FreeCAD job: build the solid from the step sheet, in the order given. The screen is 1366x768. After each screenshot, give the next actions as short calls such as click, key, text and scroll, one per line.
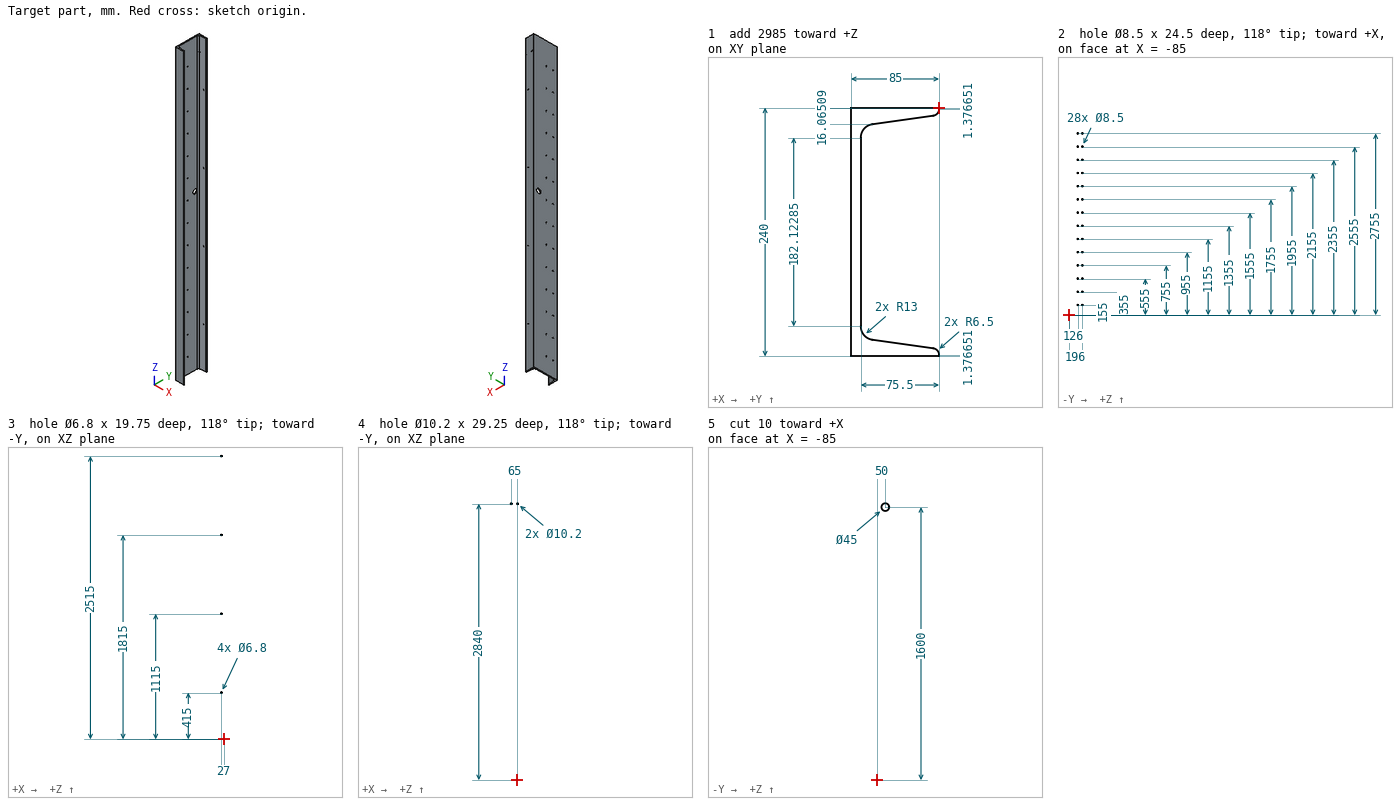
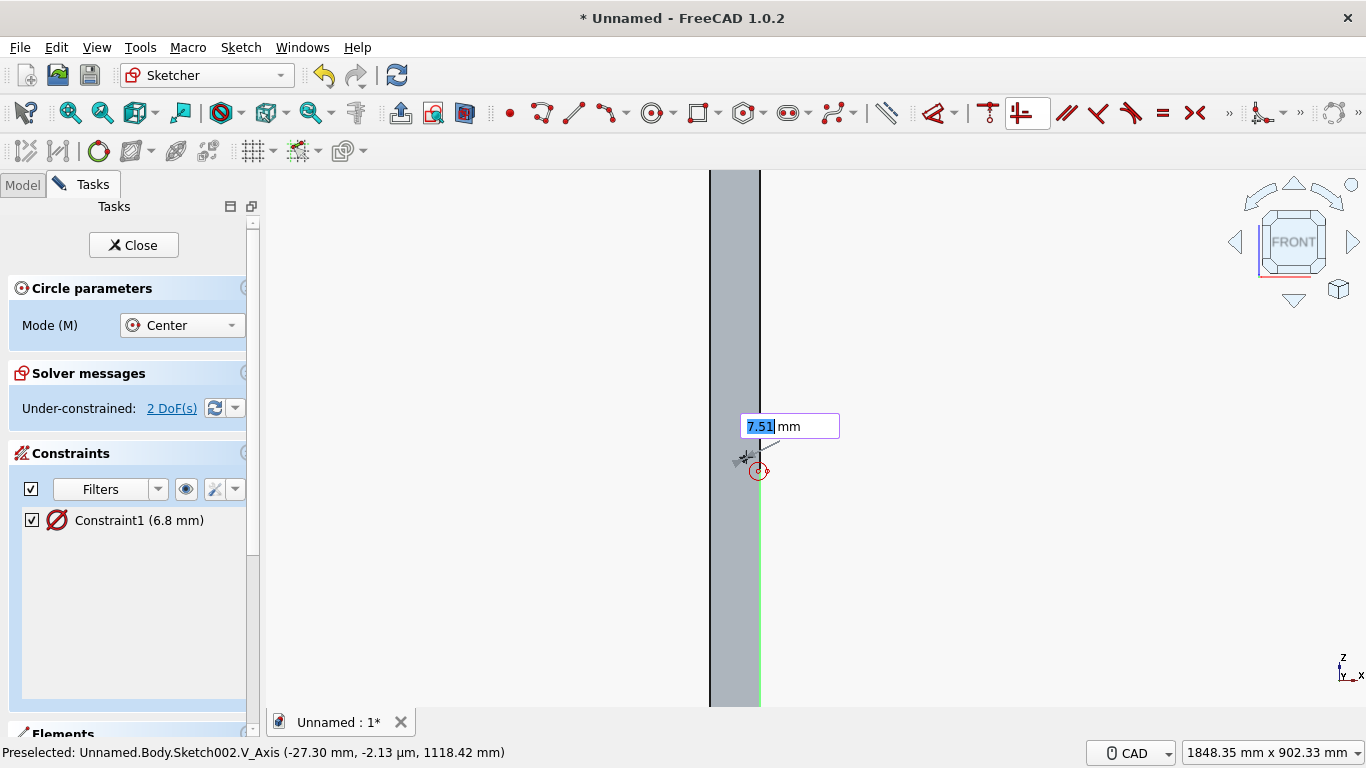
text(6.8)
key(Return)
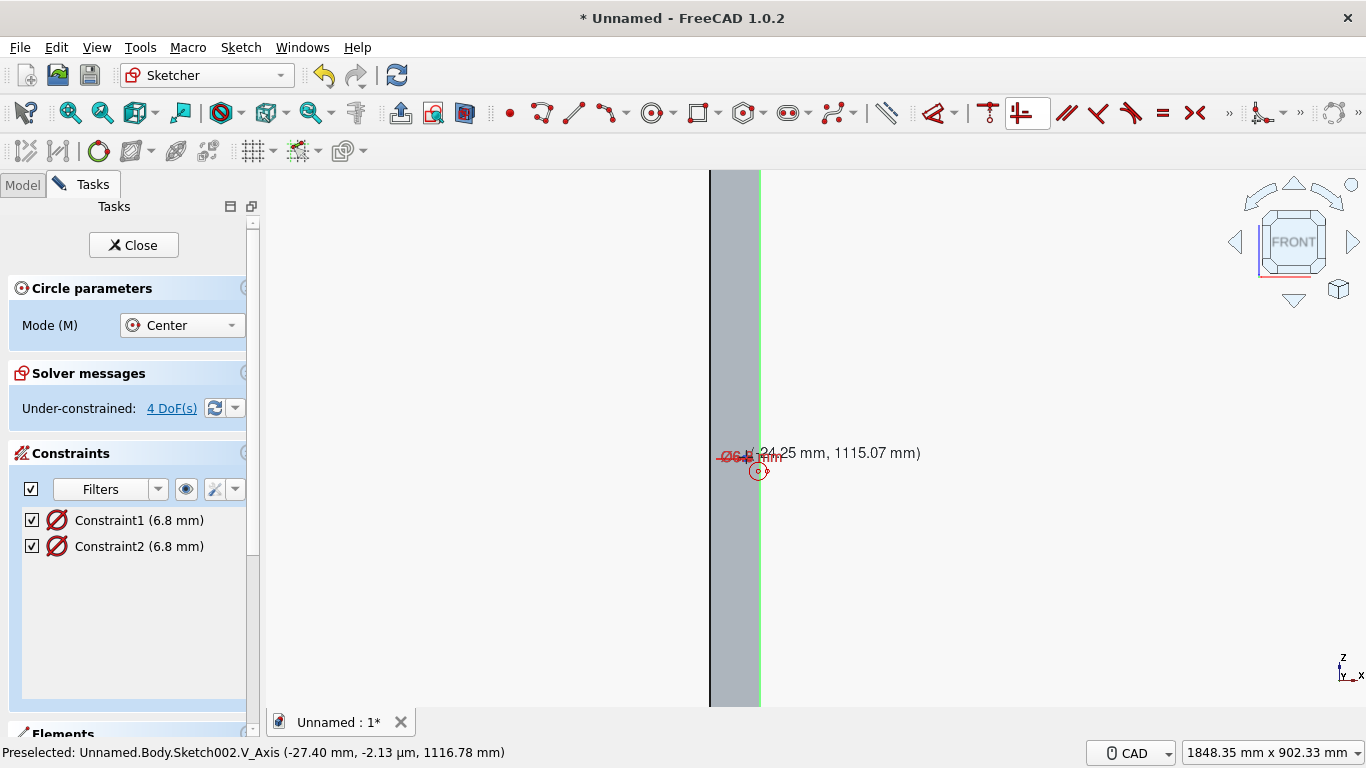
scroll(746, 460, down, 7)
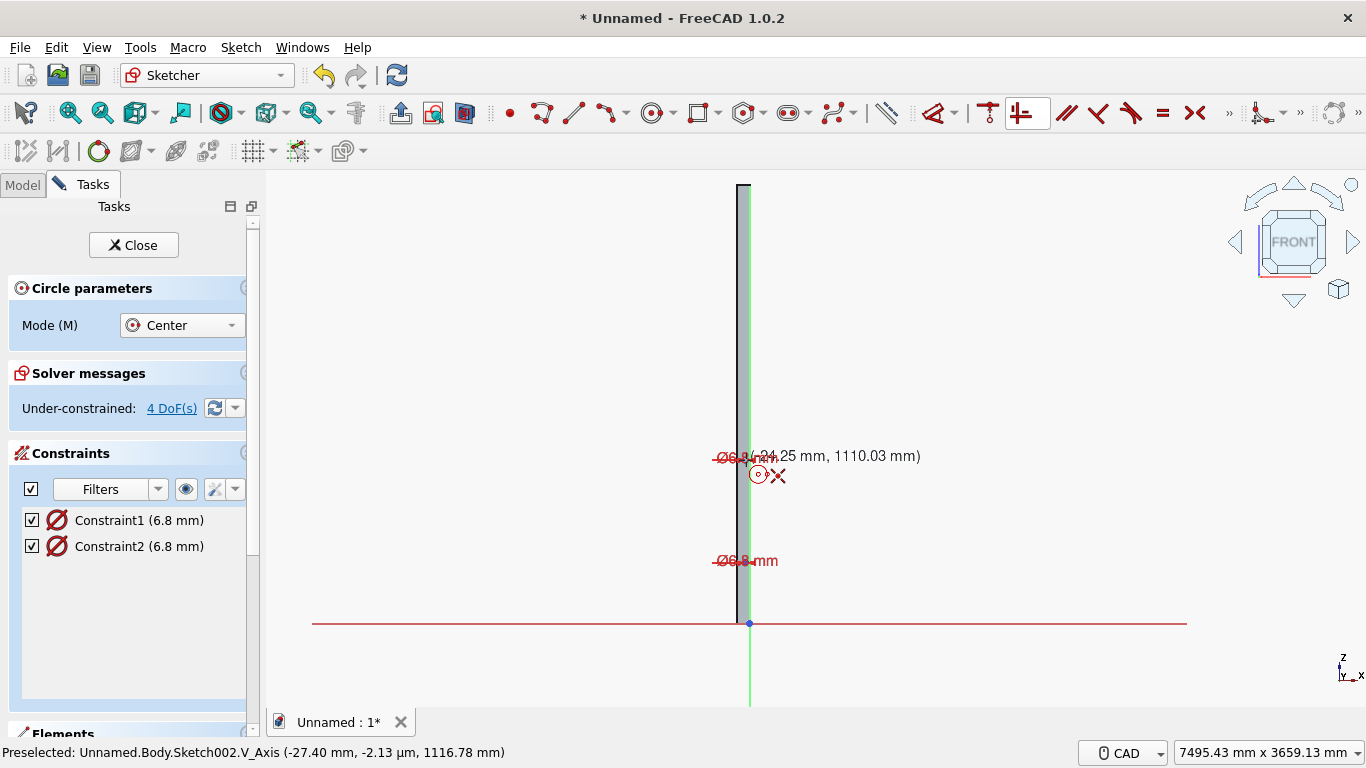
scroll(746, 357, up, 20)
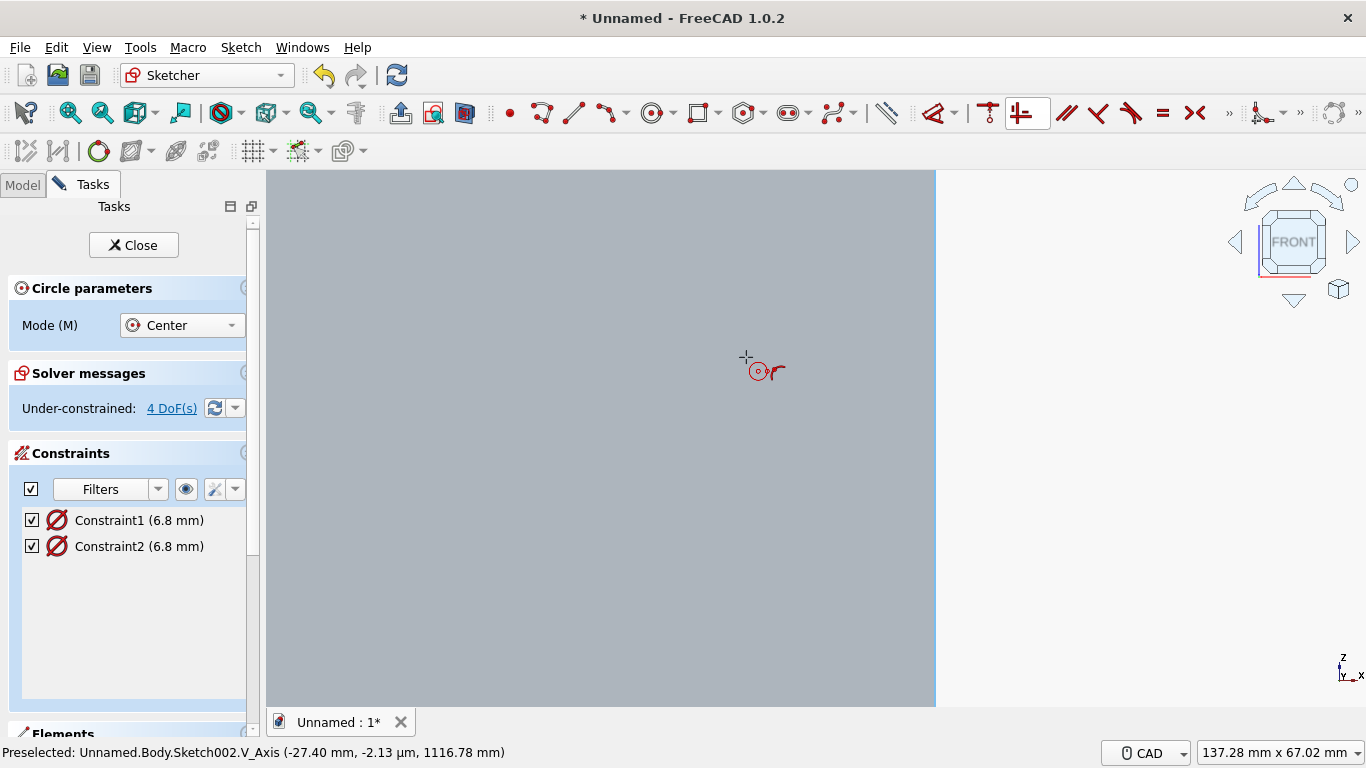
scroll(748, 438, down, 15)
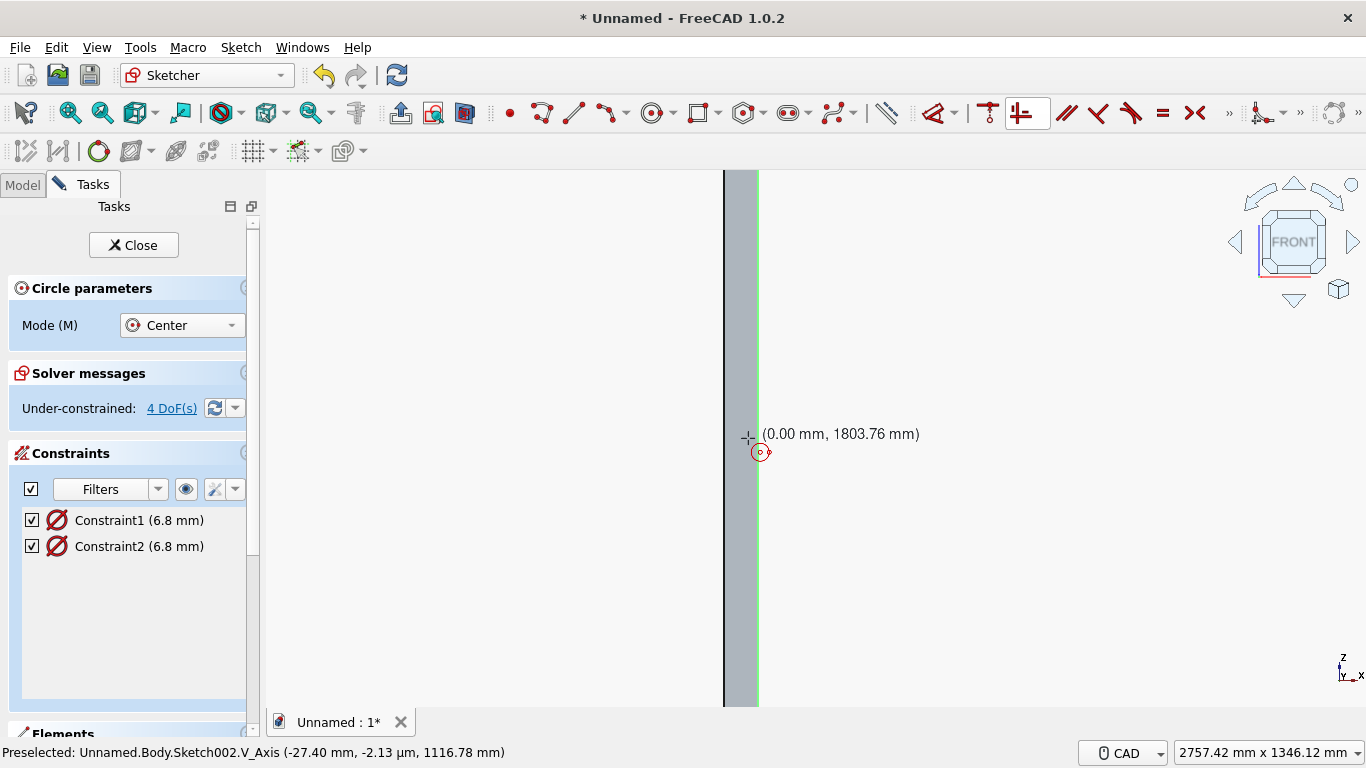
scroll(745, 312, down, 5)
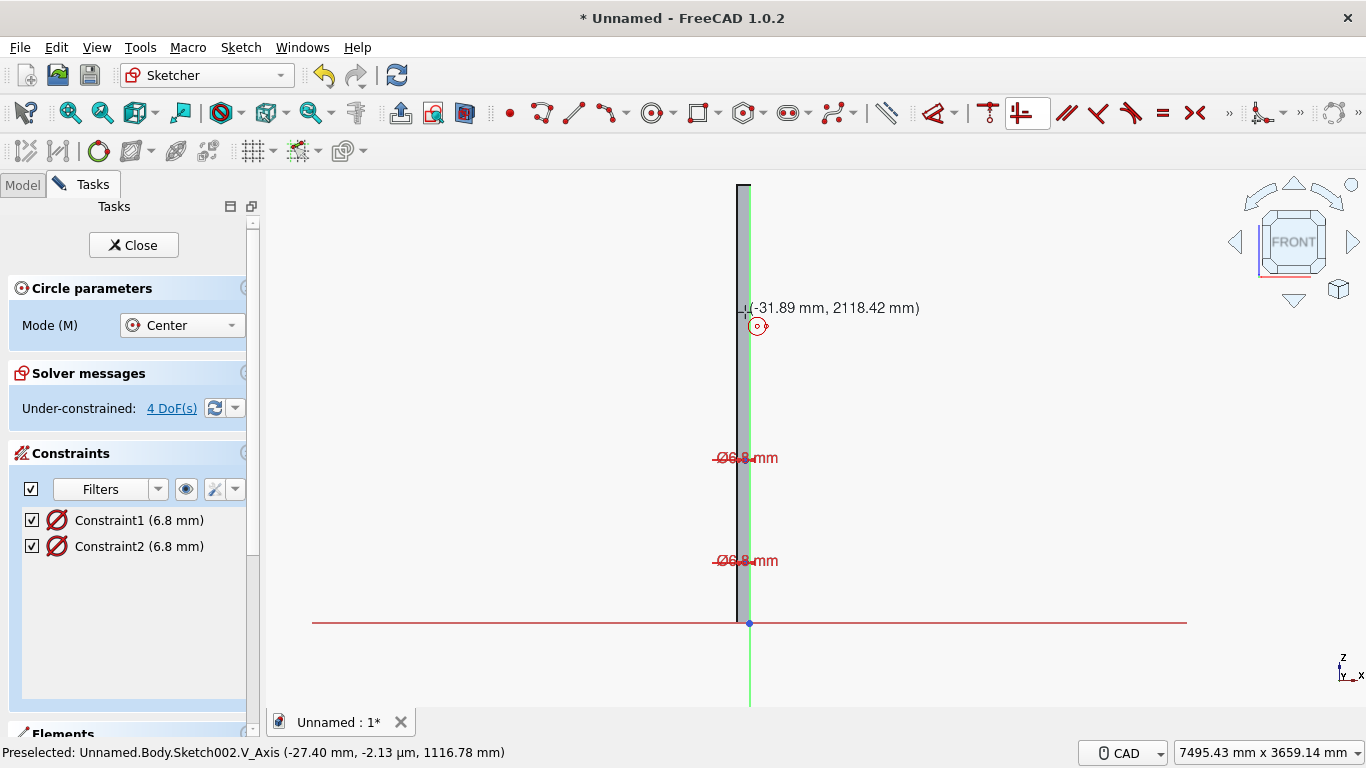
scroll(746, 357, up, 7)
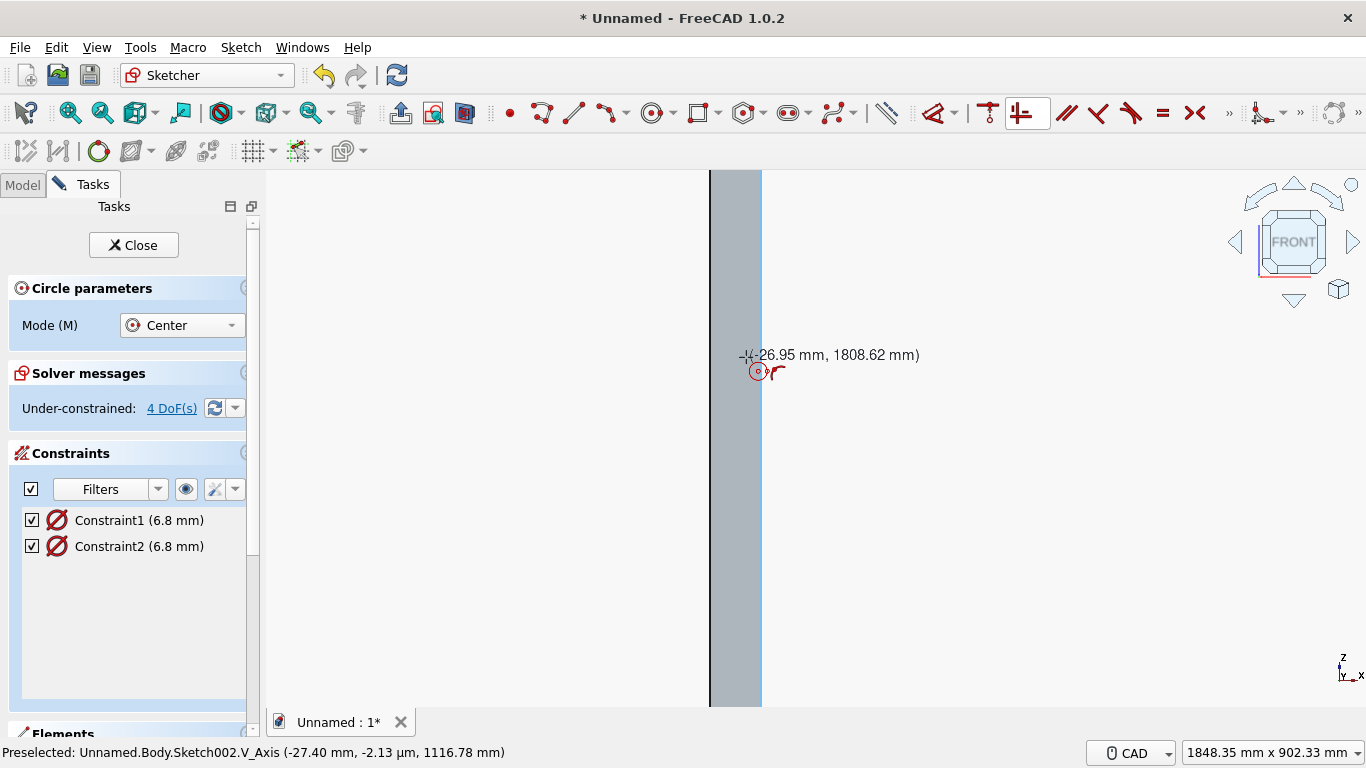
click(745, 356)
move(746, 355)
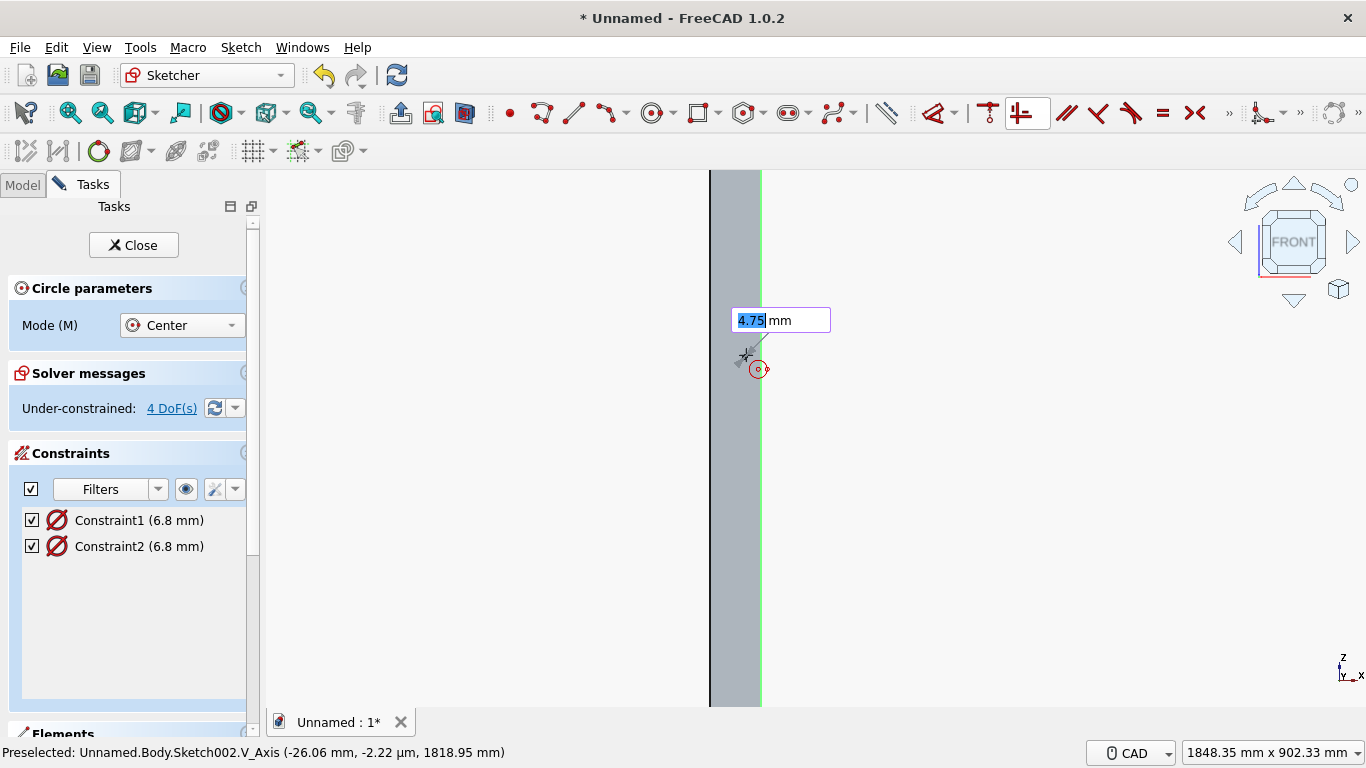
text(6.8)
key(Return)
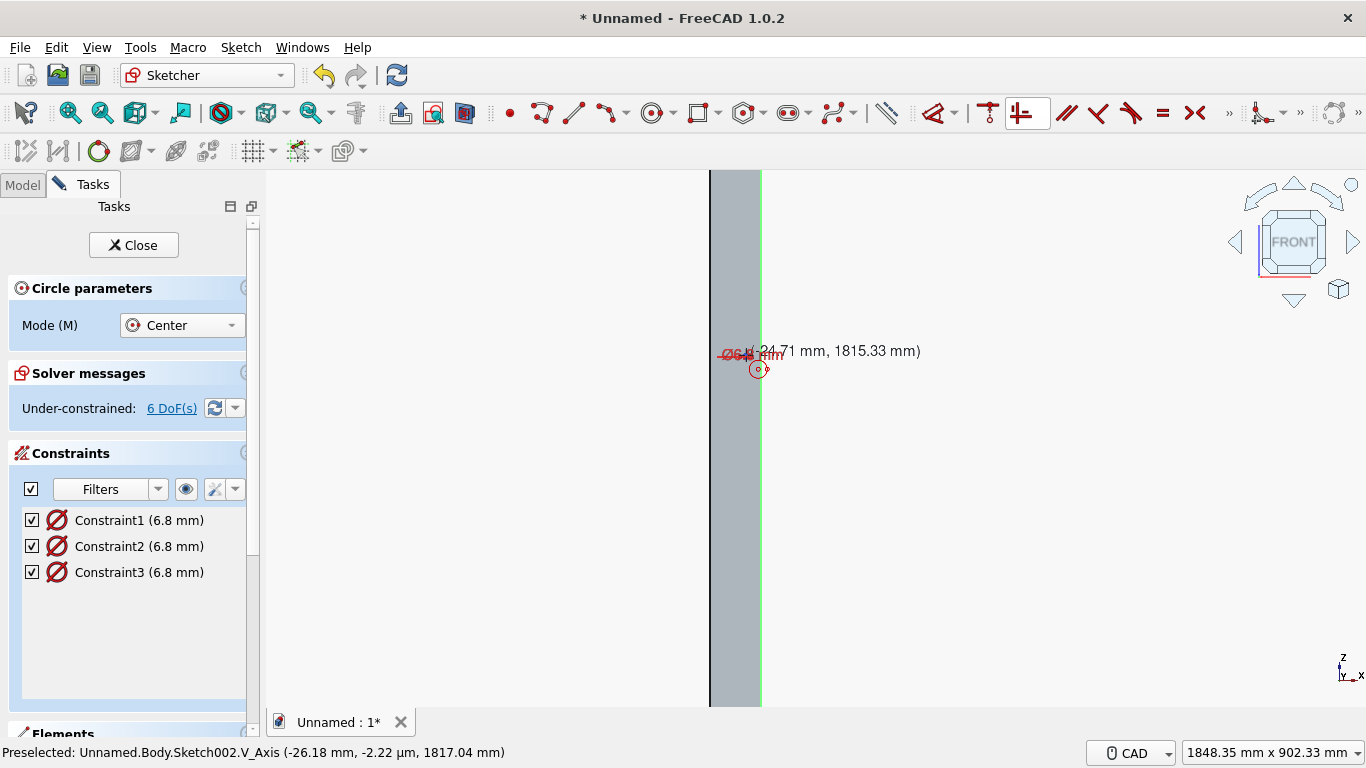
scroll(746, 357, down, 7)